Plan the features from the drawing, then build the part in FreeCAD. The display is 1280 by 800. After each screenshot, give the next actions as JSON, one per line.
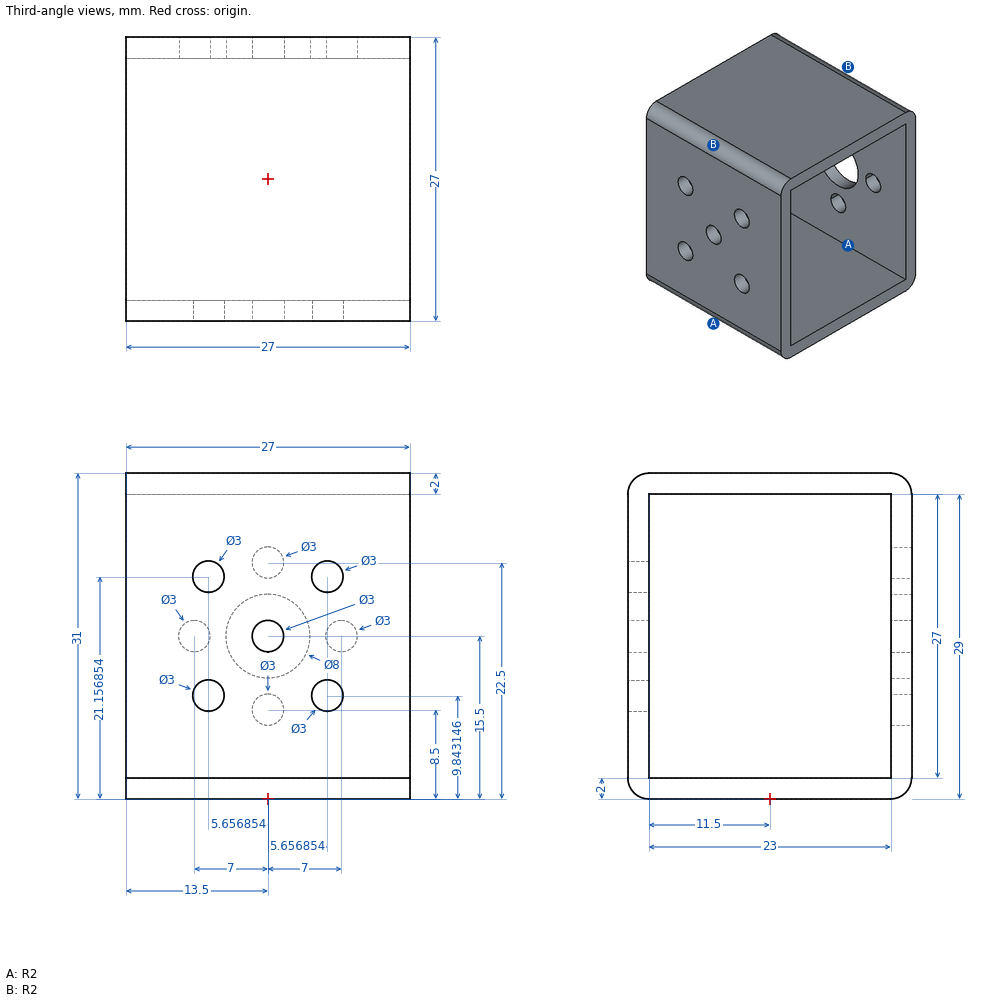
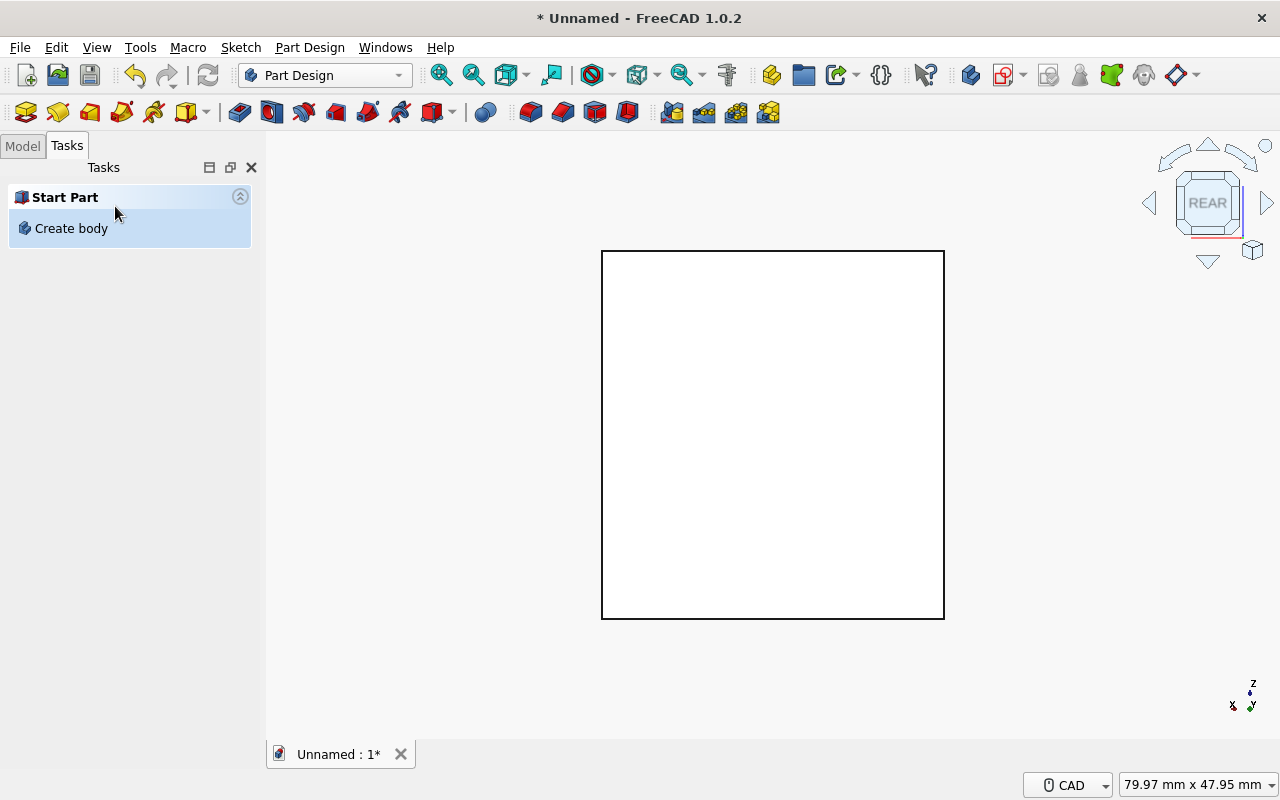
{"action": "left_click", "coordinate": [773, 434]}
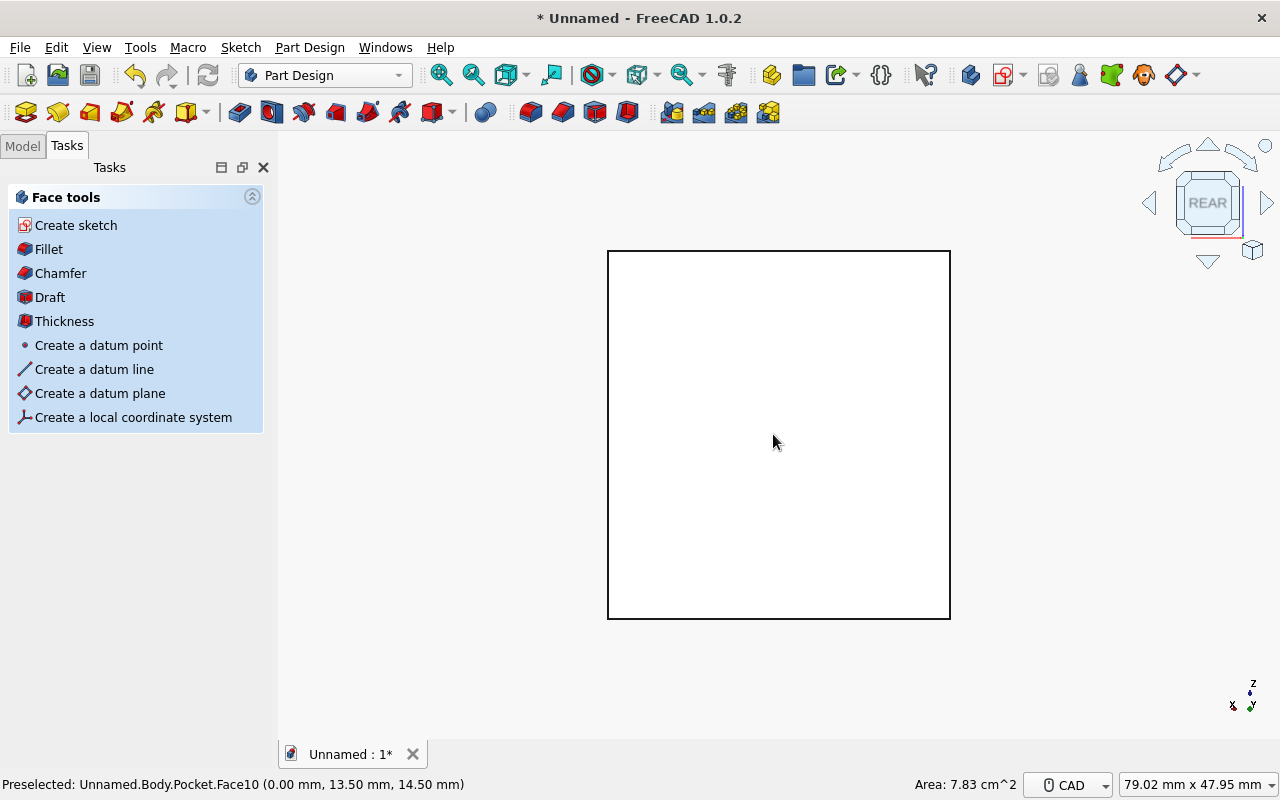
{"action": "left_click", "coordinate": [1004, 76]}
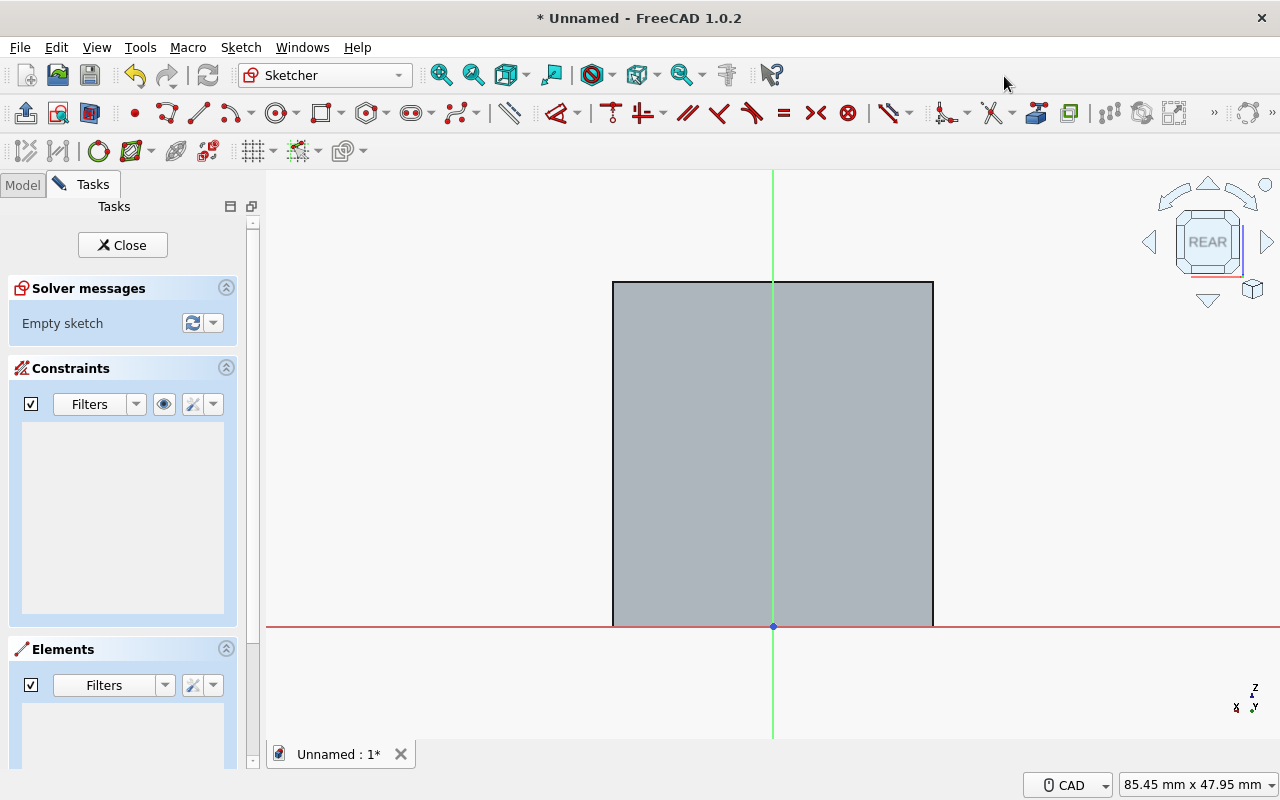
{"action": "scroll", "coordinate": [912, 625], "scroll_direction": "up", "scroll_amount": 2}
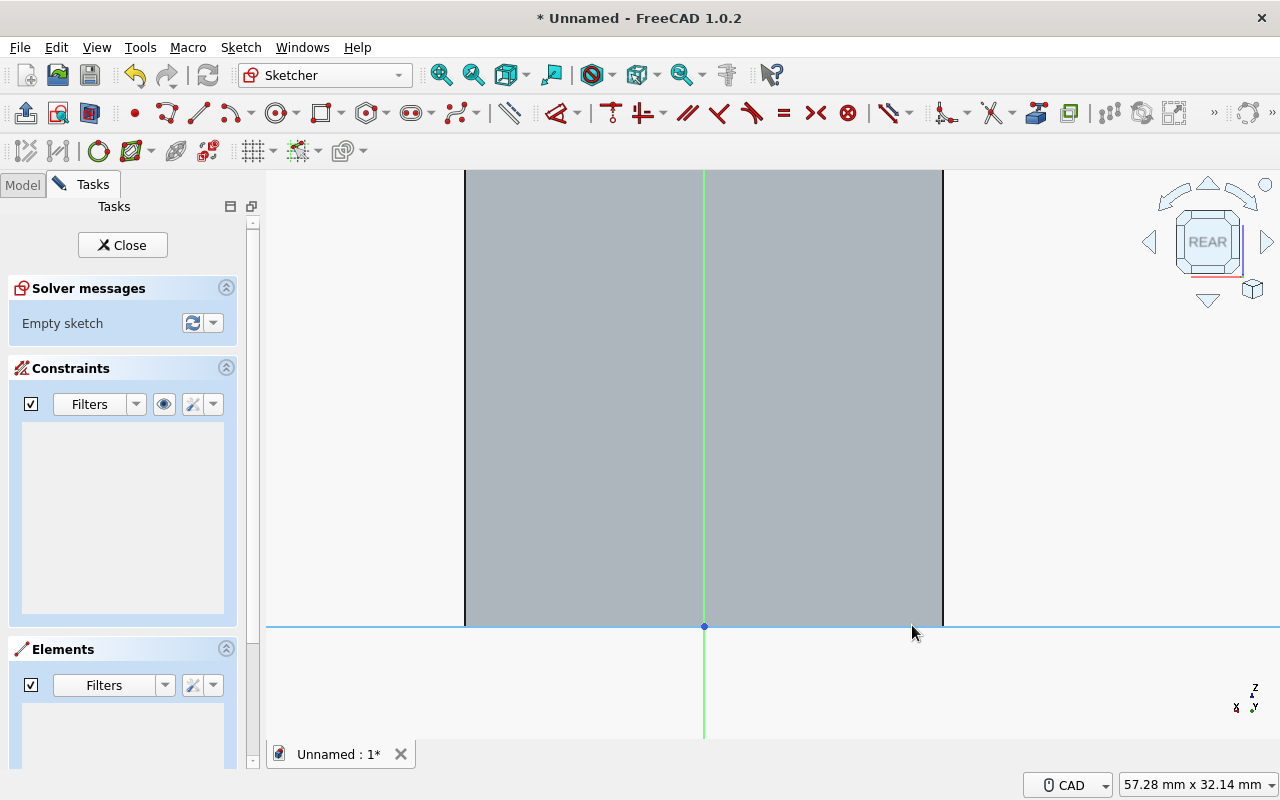
{"action": "left_click", "coordinate": [276, 114]}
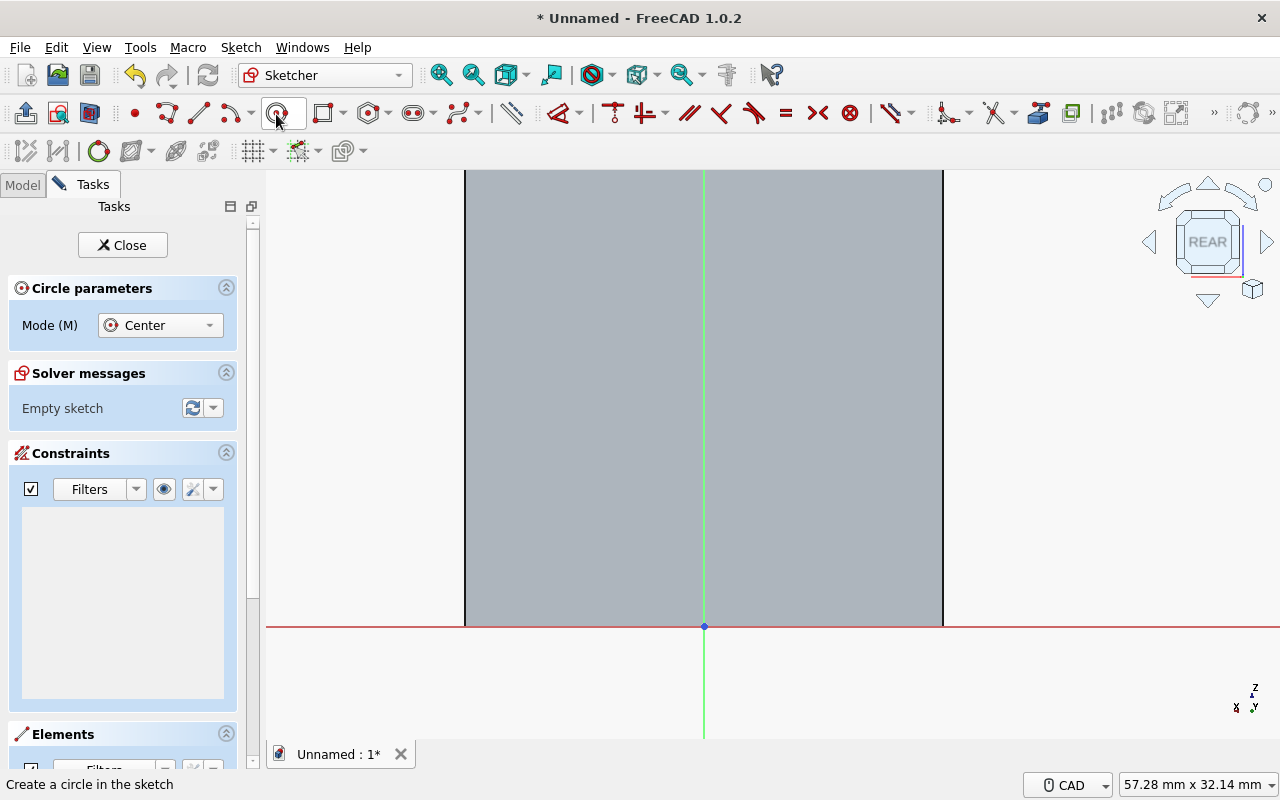
{"action": "left_click", "coordinate": [704, 353]}
{"action": "mouse_move", "coordinate": [754, 302]}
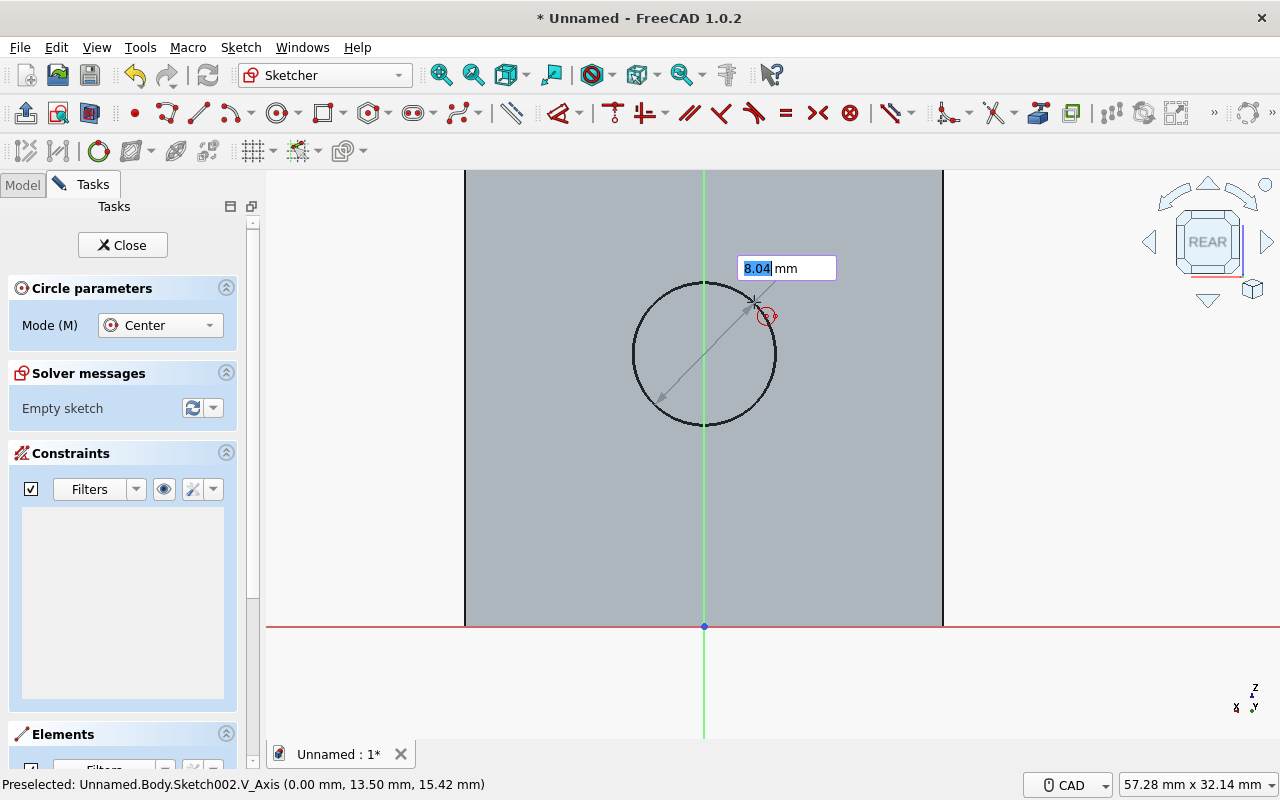
{"action": "type", "text": "8"}
{"action": "key", "text": "Return"}
{"action": "key", "text": "Escape"}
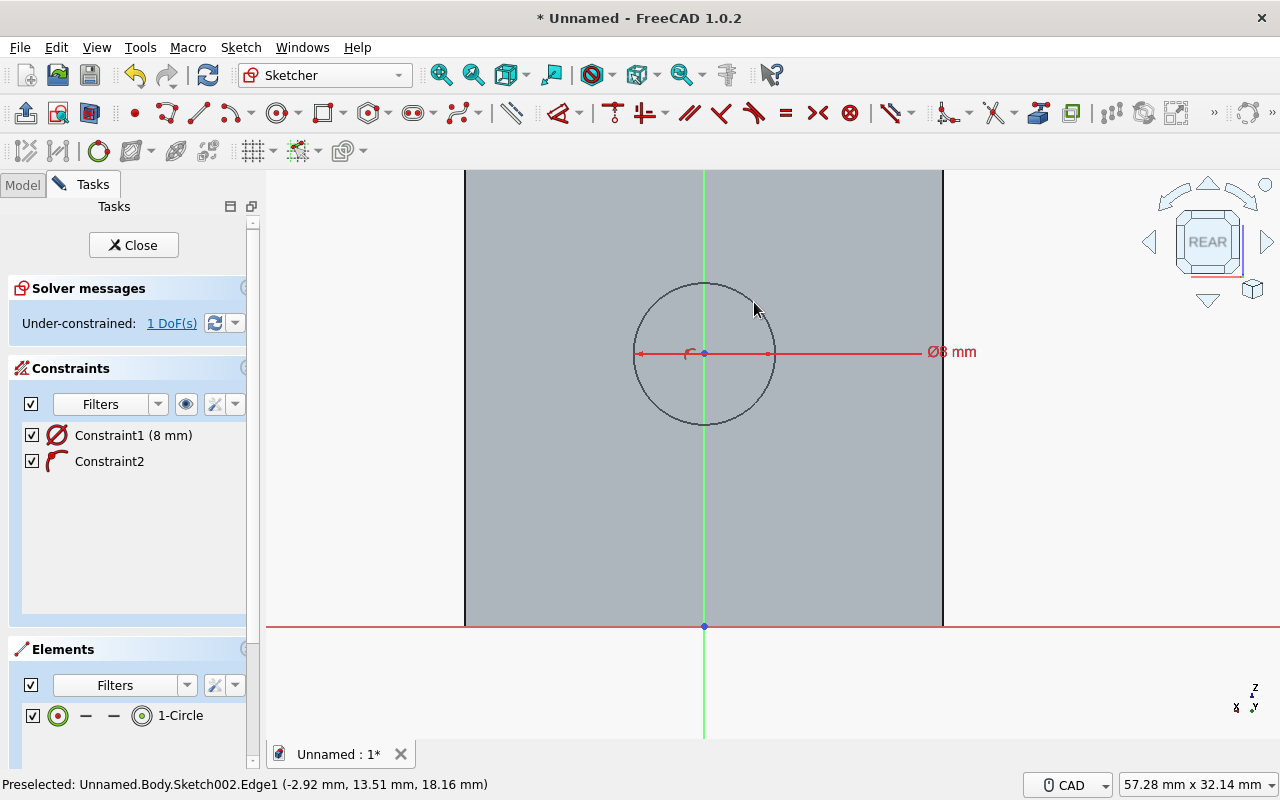
{"action": "left_click", "coordinate": [558, 114]}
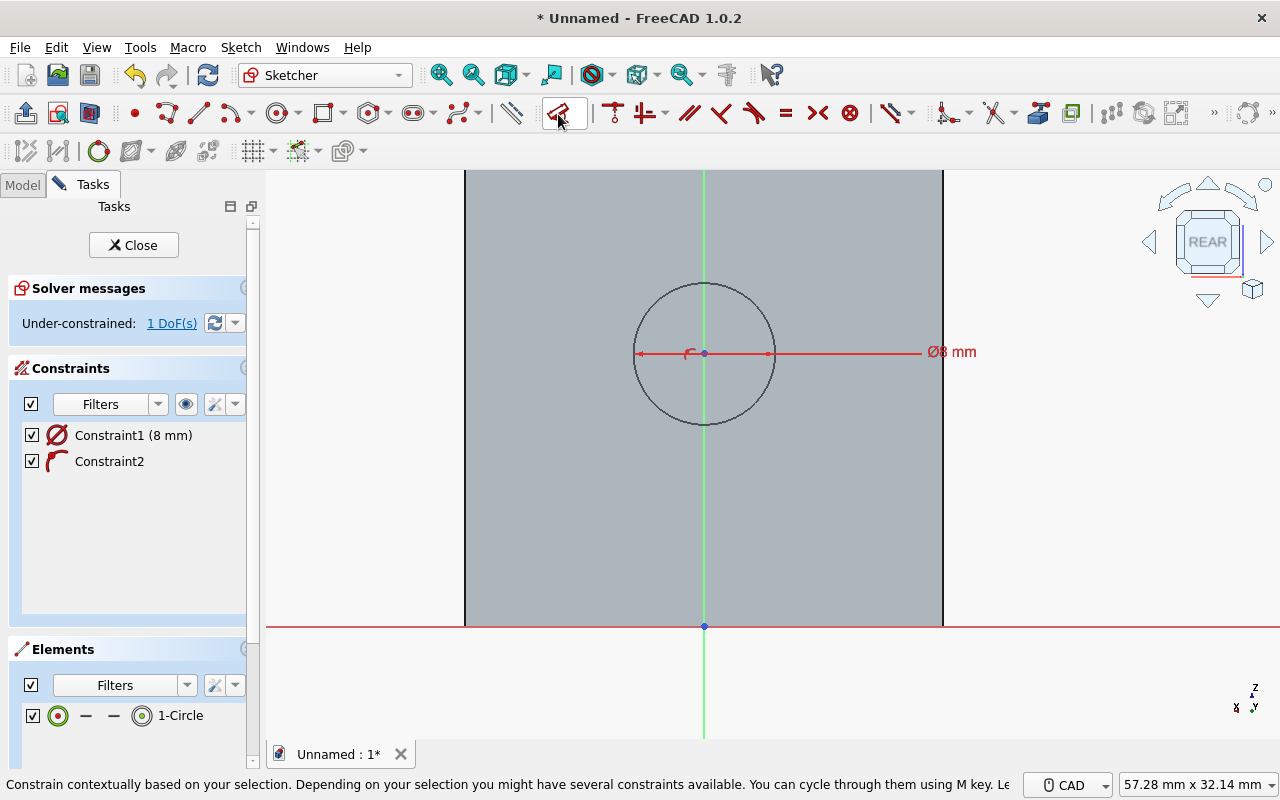
{"action": "left_click", "coordinate": [704, 354]}
{"action": "left_click", "coordinate": [738, 490]}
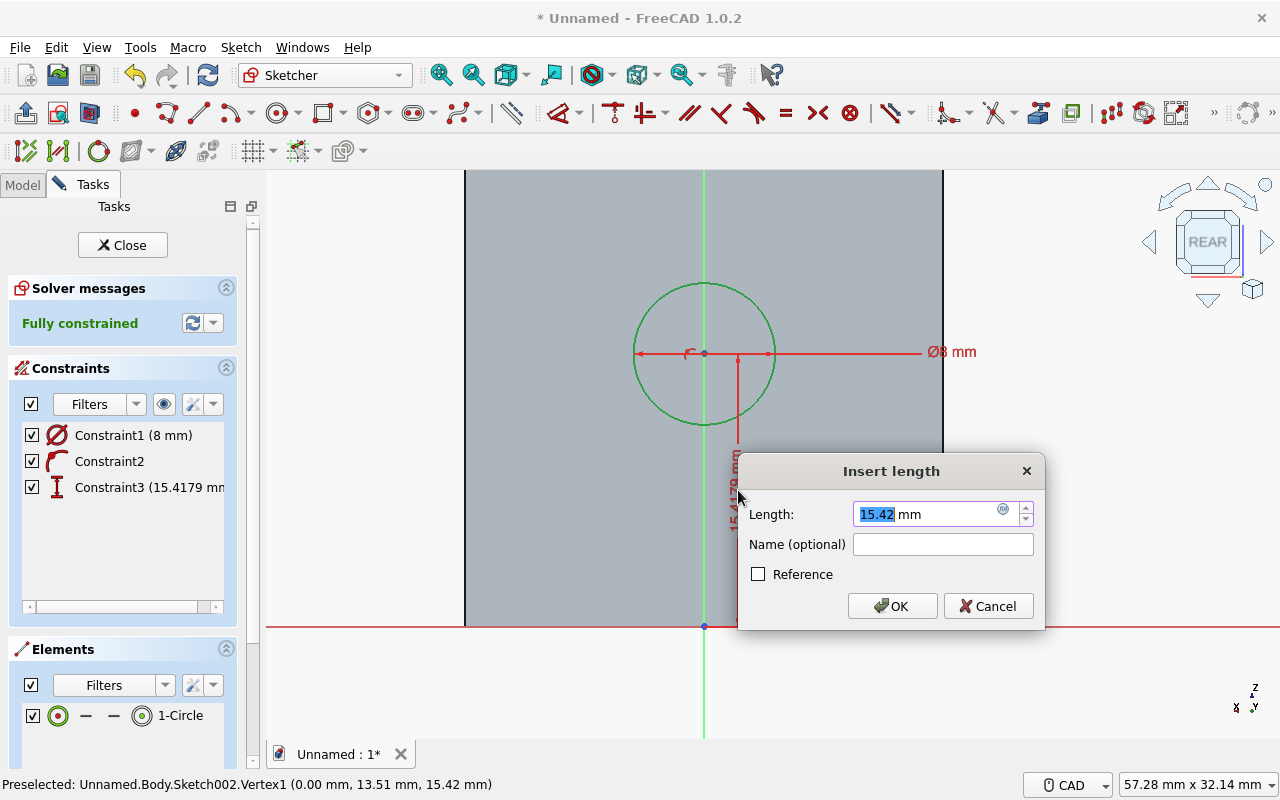
{"action": "type", "text": "15.5"}
{"action": "key", "text": "Return"}
{"action": "key", "text": "Escape"}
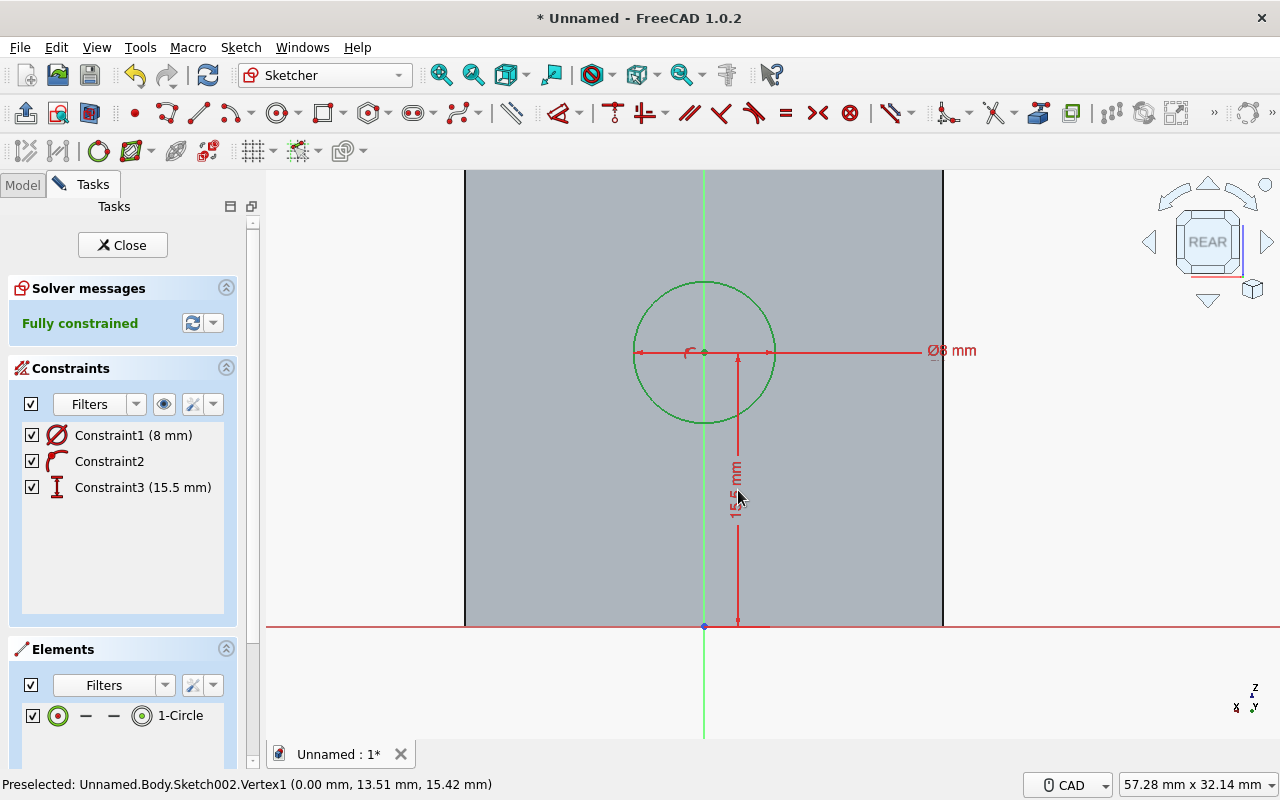
{"action": "left_click", "coordinate": [123, 245]}